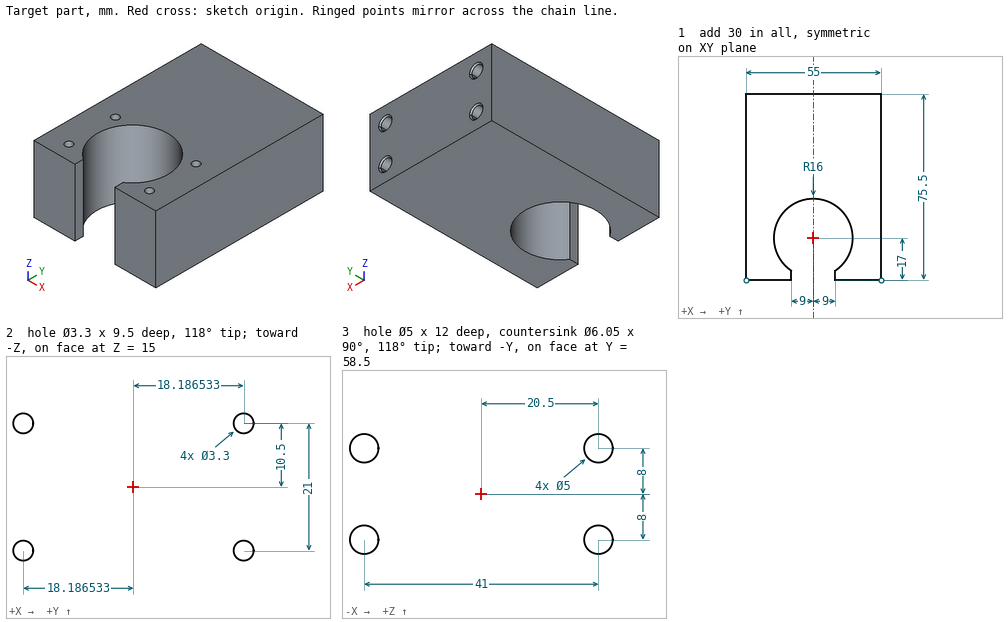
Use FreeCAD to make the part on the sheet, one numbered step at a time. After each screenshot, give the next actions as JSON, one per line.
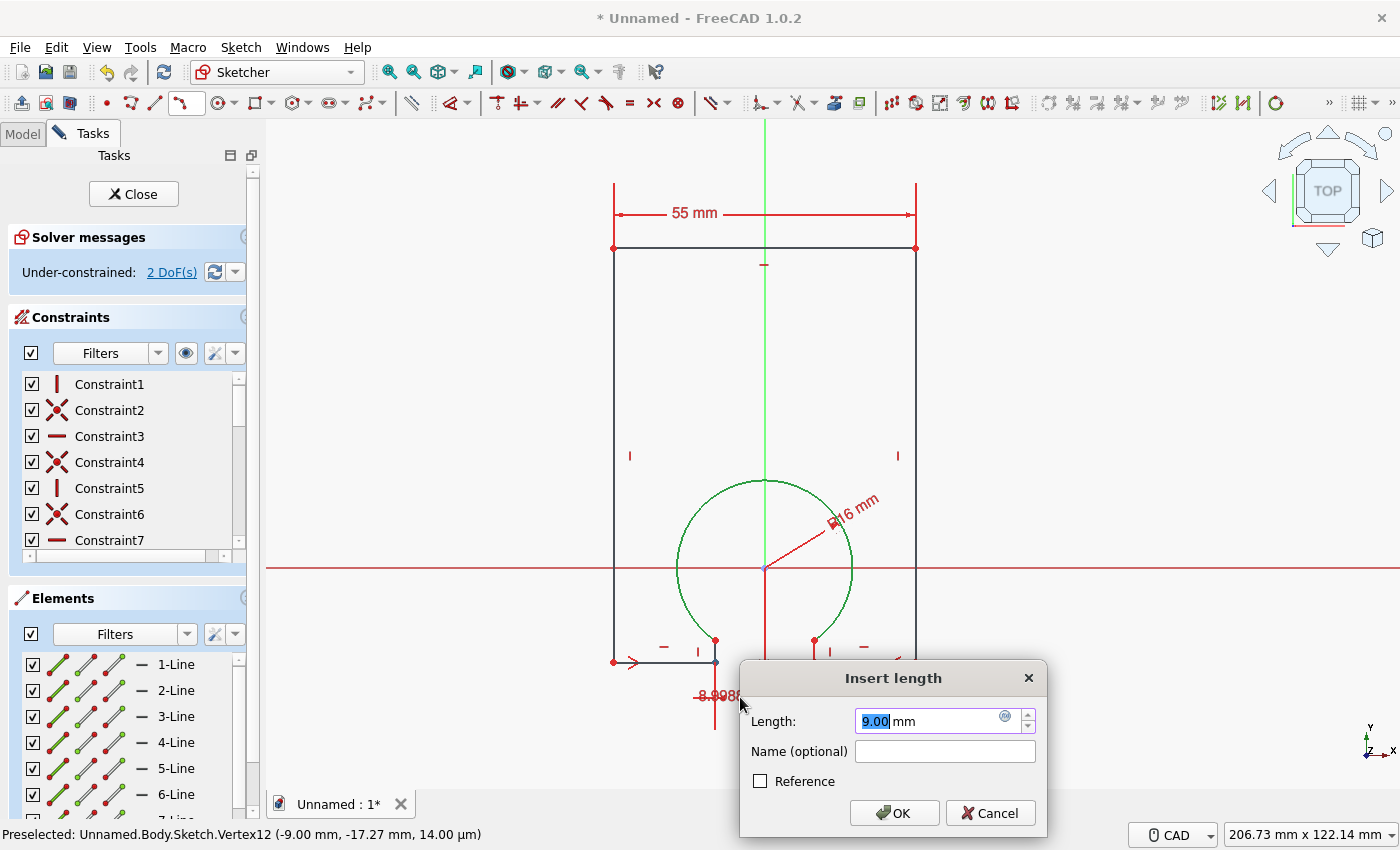
{"action": "type", "text": "9"}
{"action": "key", "text": "Return"}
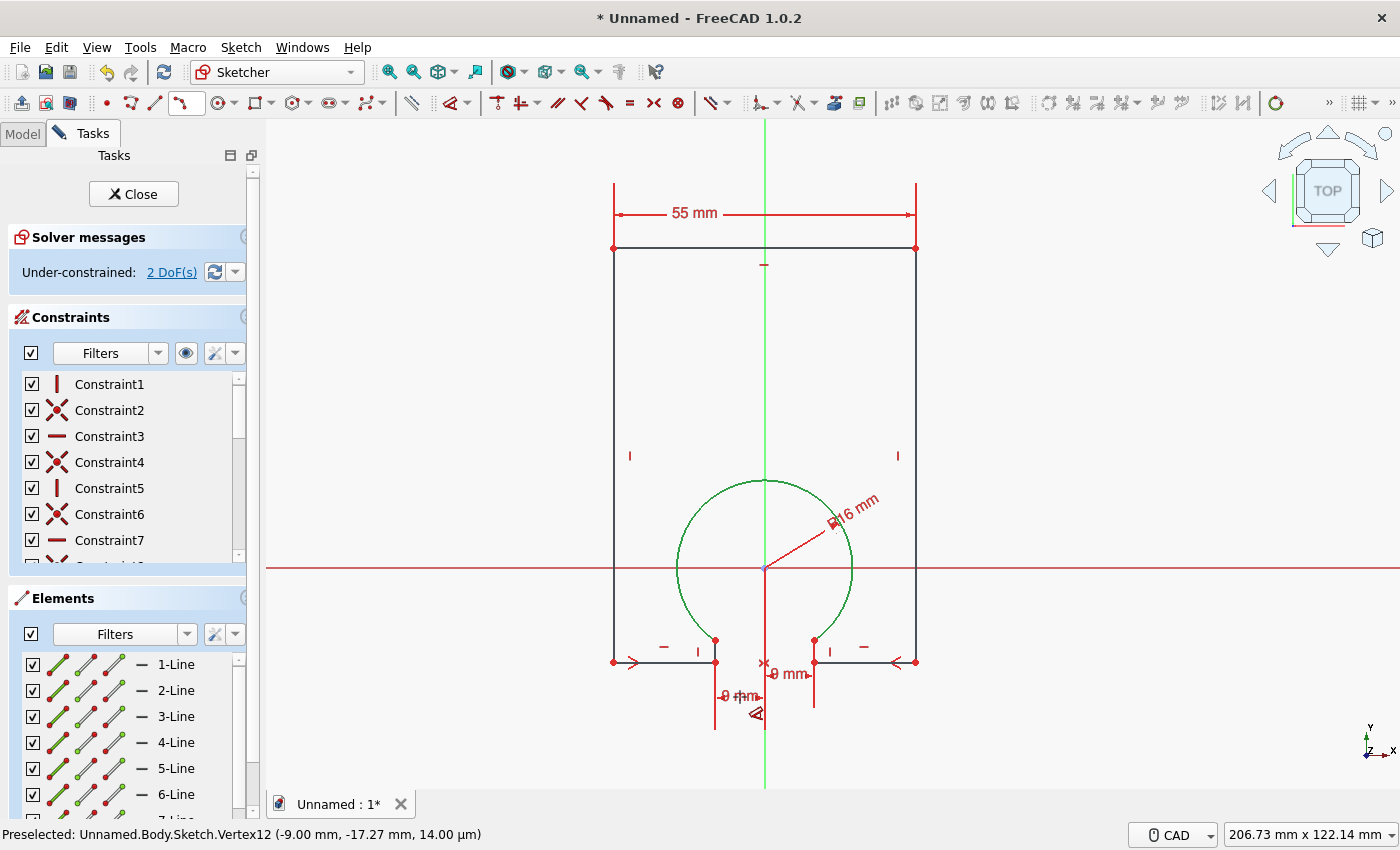
{"action": "left_click", "coordinate": [814, 663]}
{"action": "left_click", "coordinate": [848, 637]}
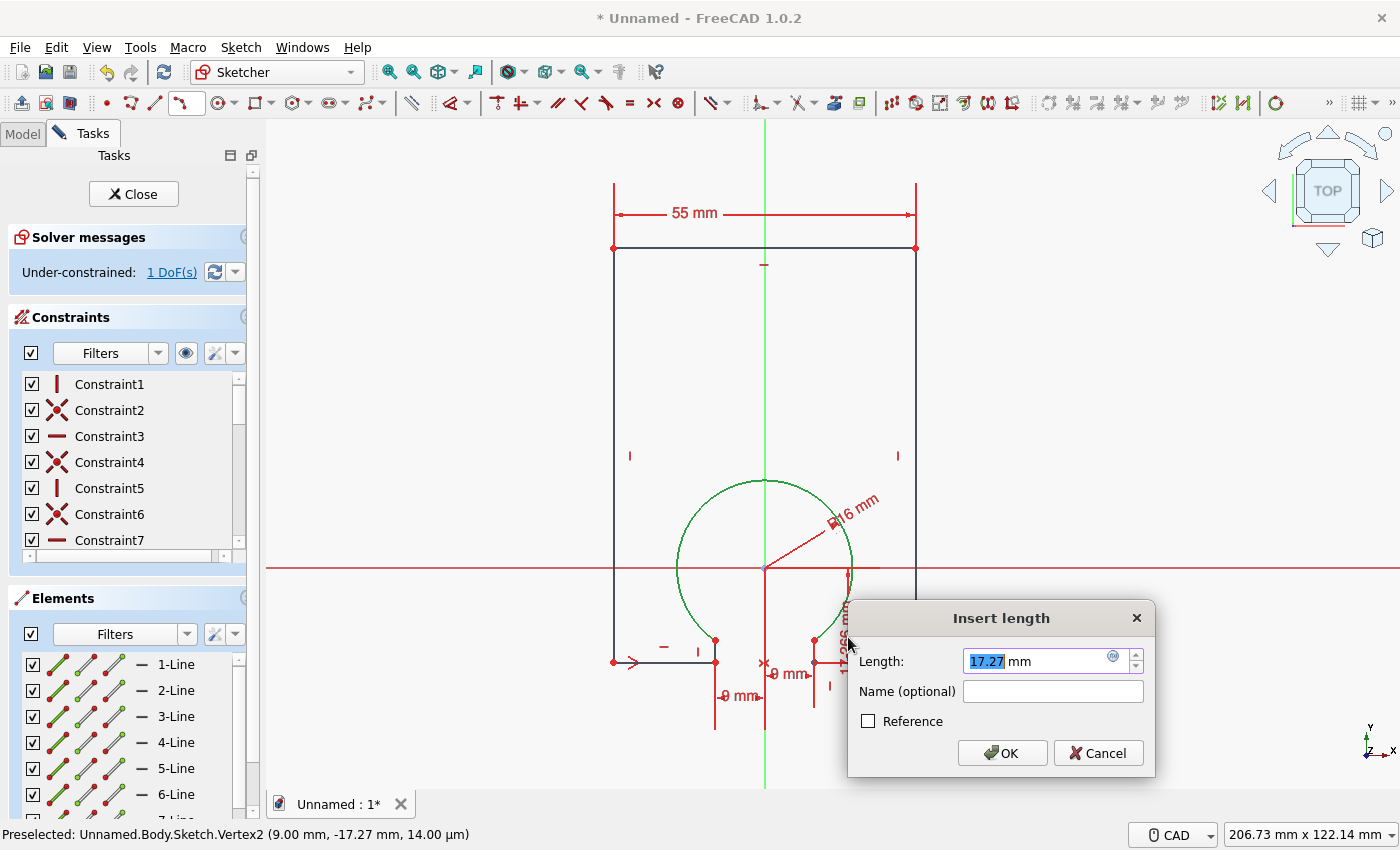
{"action": "type", "text": "17"}
{"action": "key", "text": "Return"}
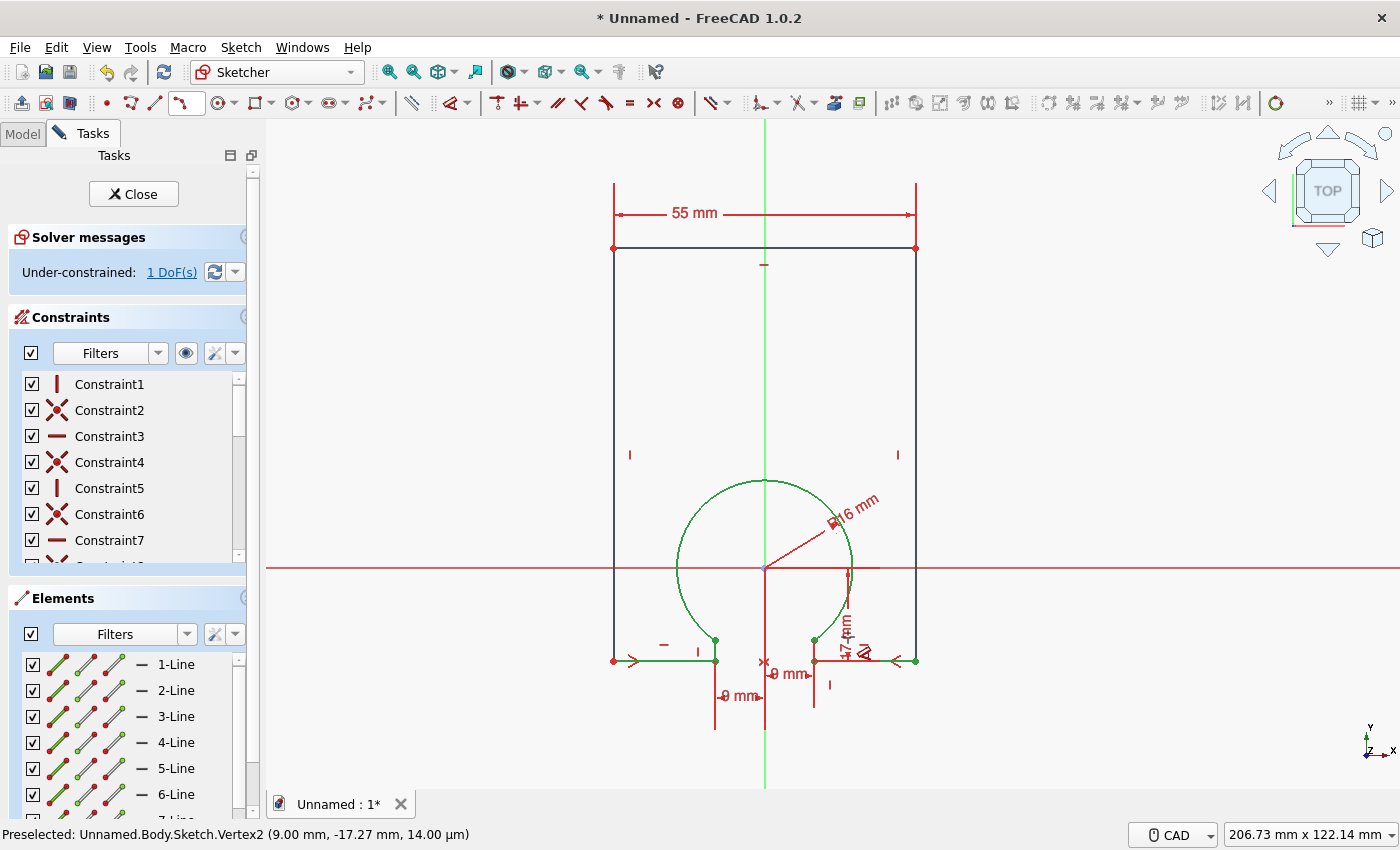
{"action": "left_click", "coordinate": [916, 537]}
{"action": "left_click", "coordinate": [950, 455]}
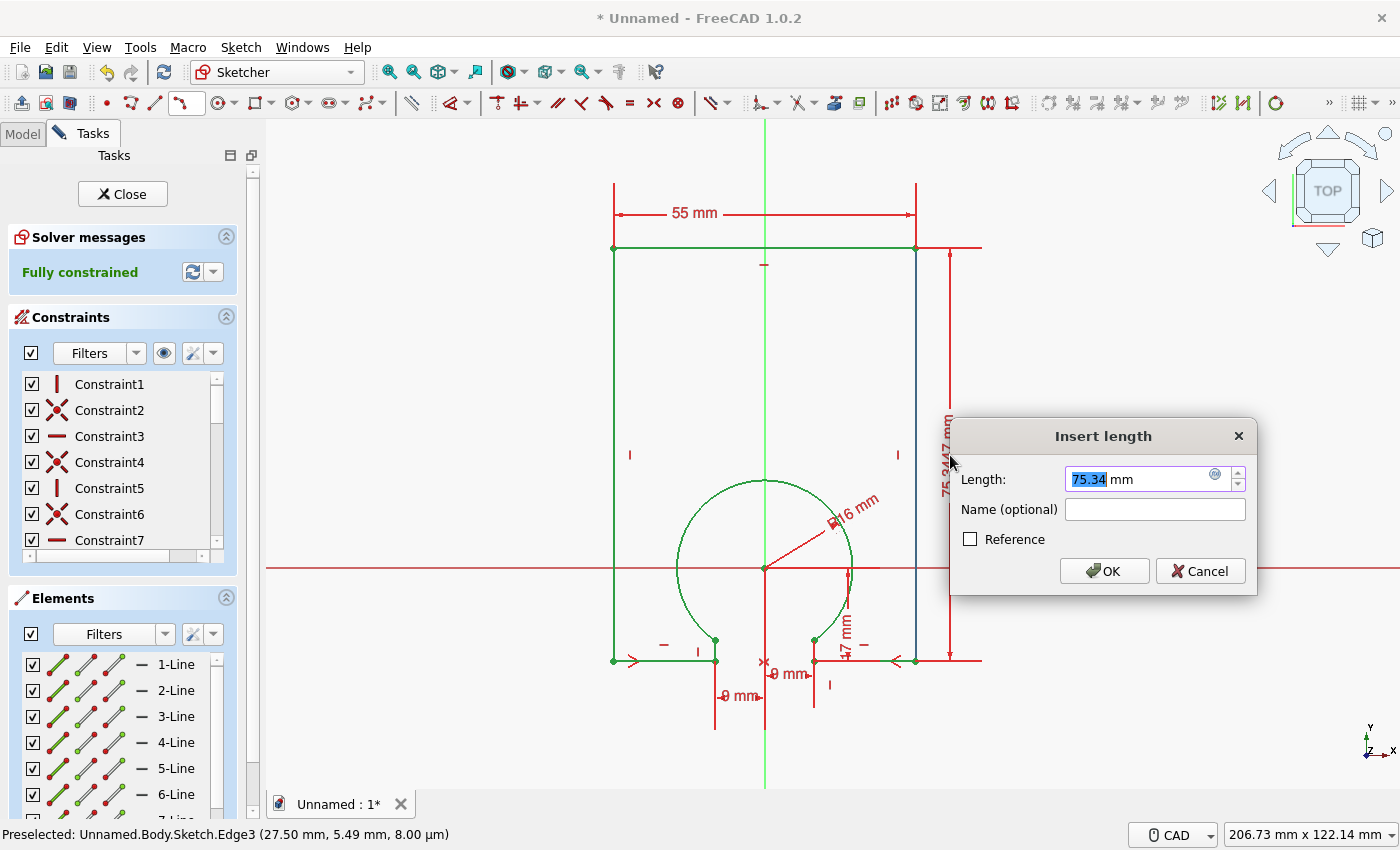
{"action": "type", "text": "75.5"}
{"action": "key", "text": "Return"}
{"action": "key", "text": "Escape"}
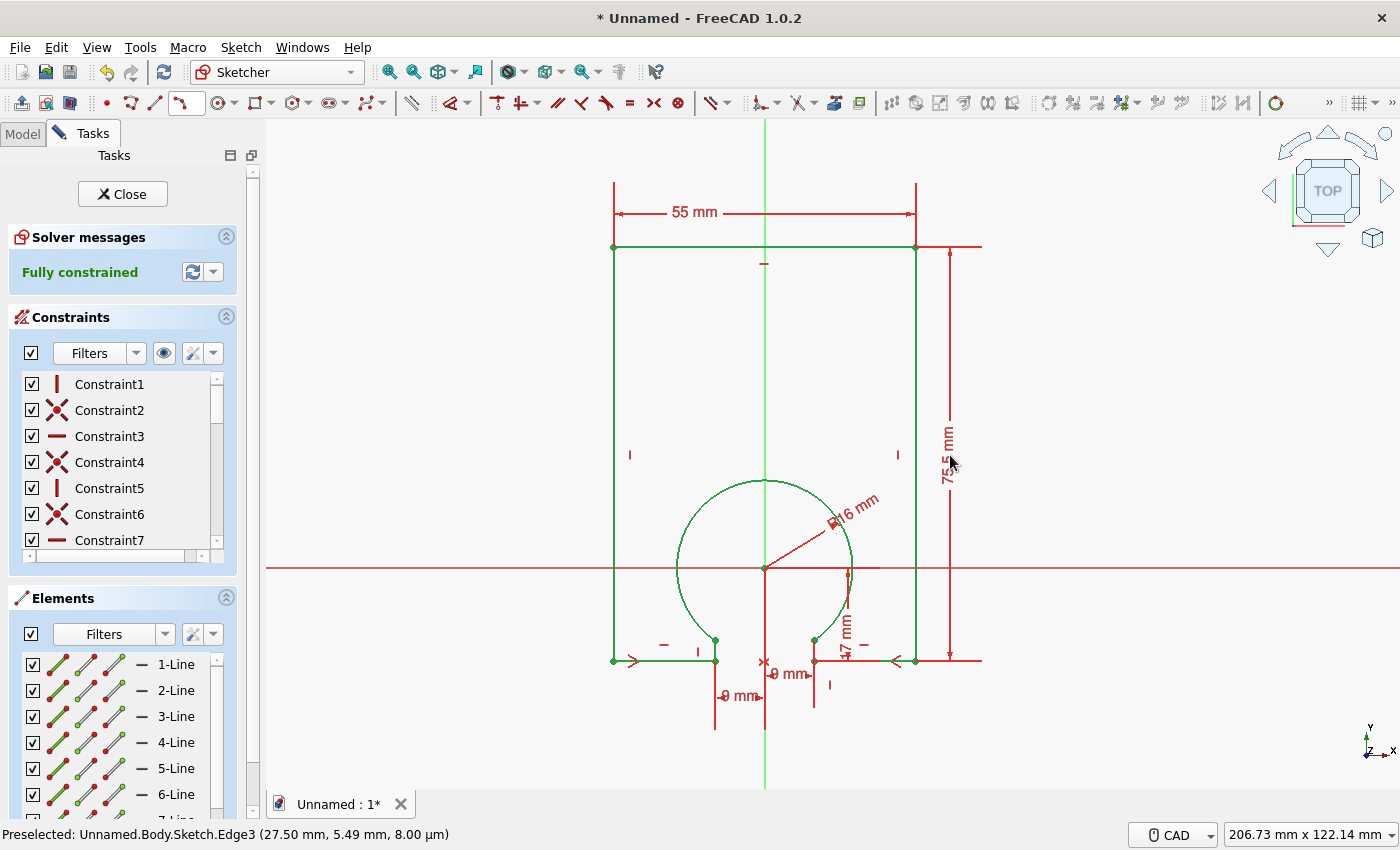
{"action": "left_click", "coordinate": [123, 194]}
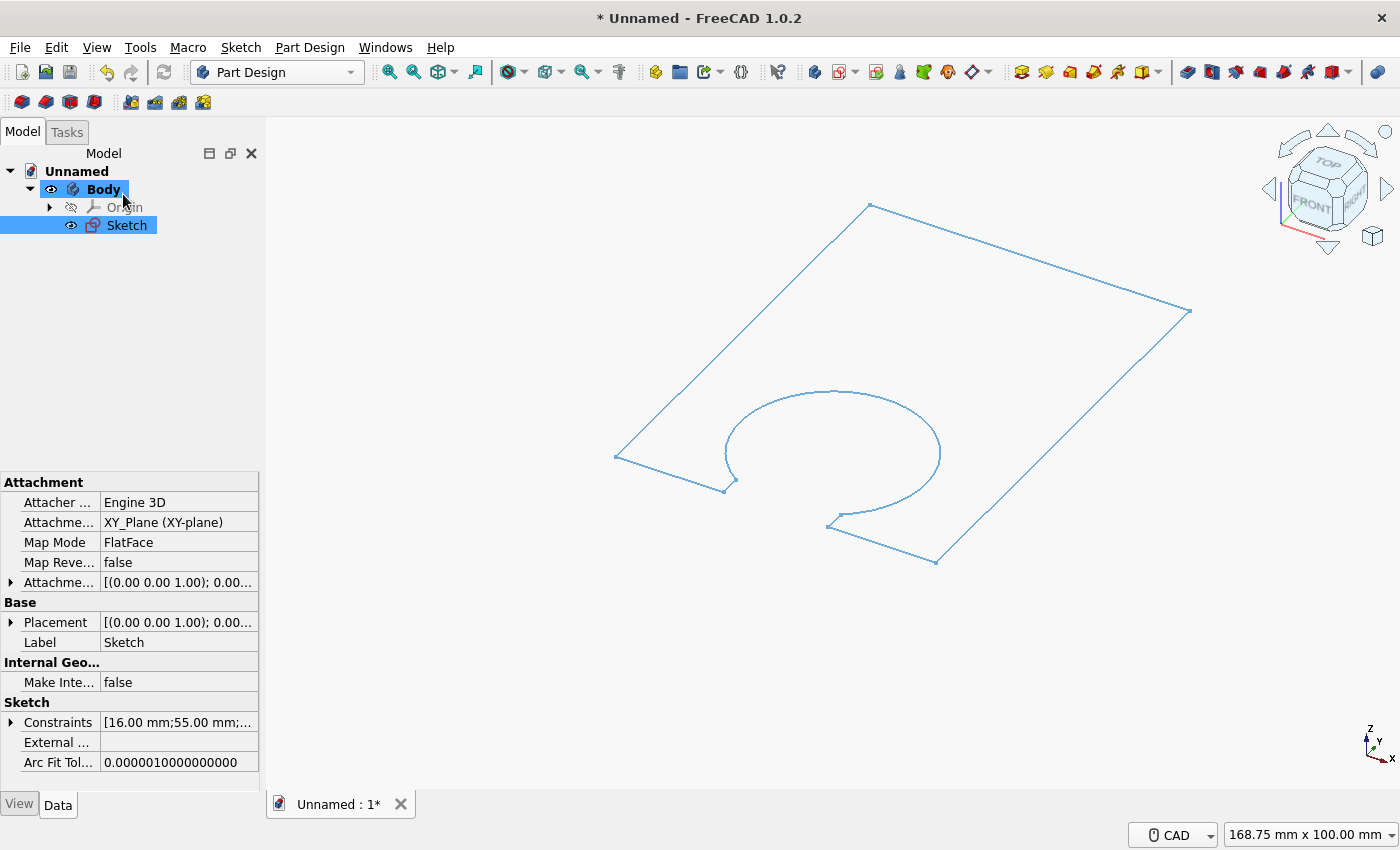
{"action": "left_click", "coordinate": [1022, 72]}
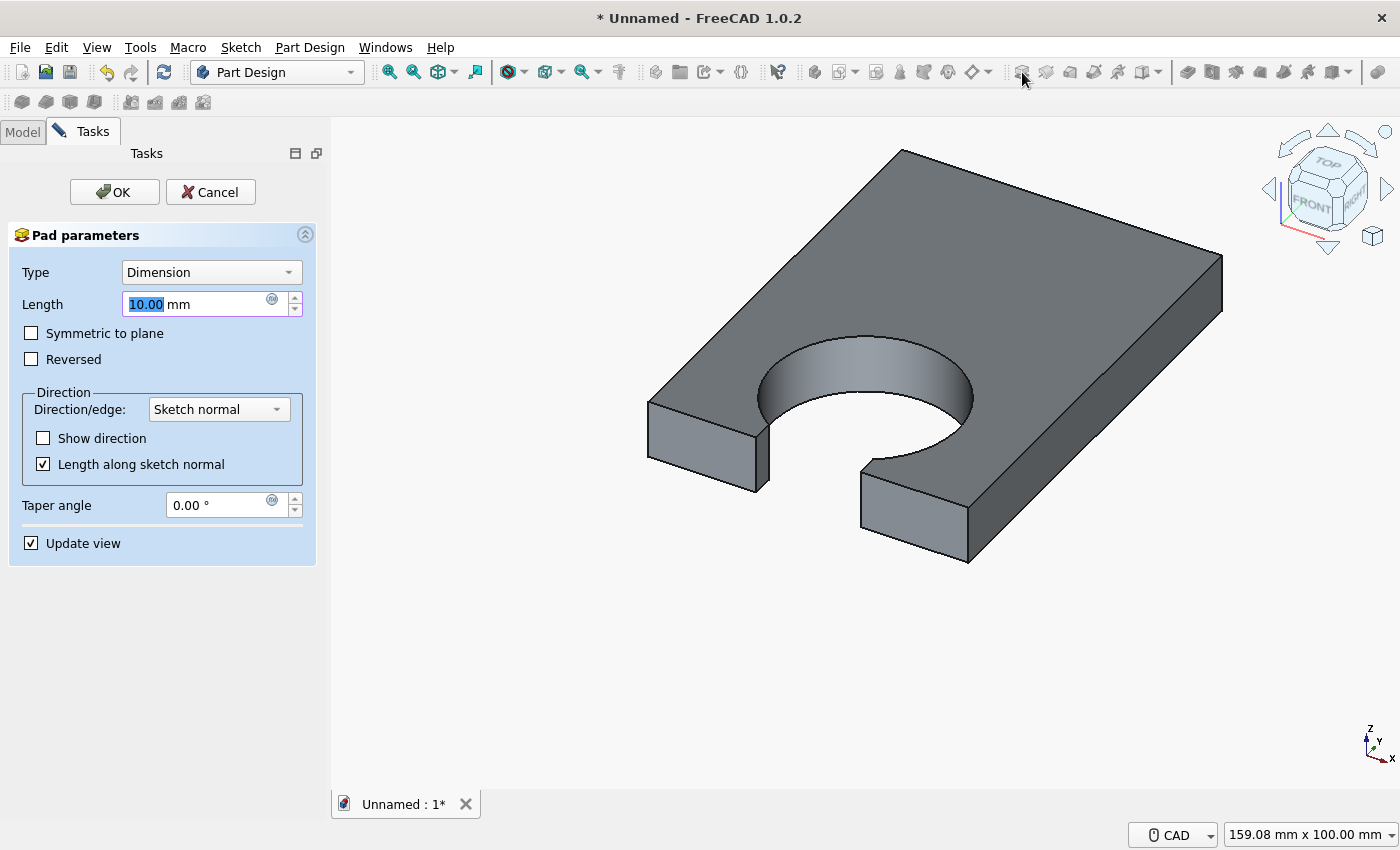
{"action": "type", "text": "30"}
{"action": "key", "text": "Tab"}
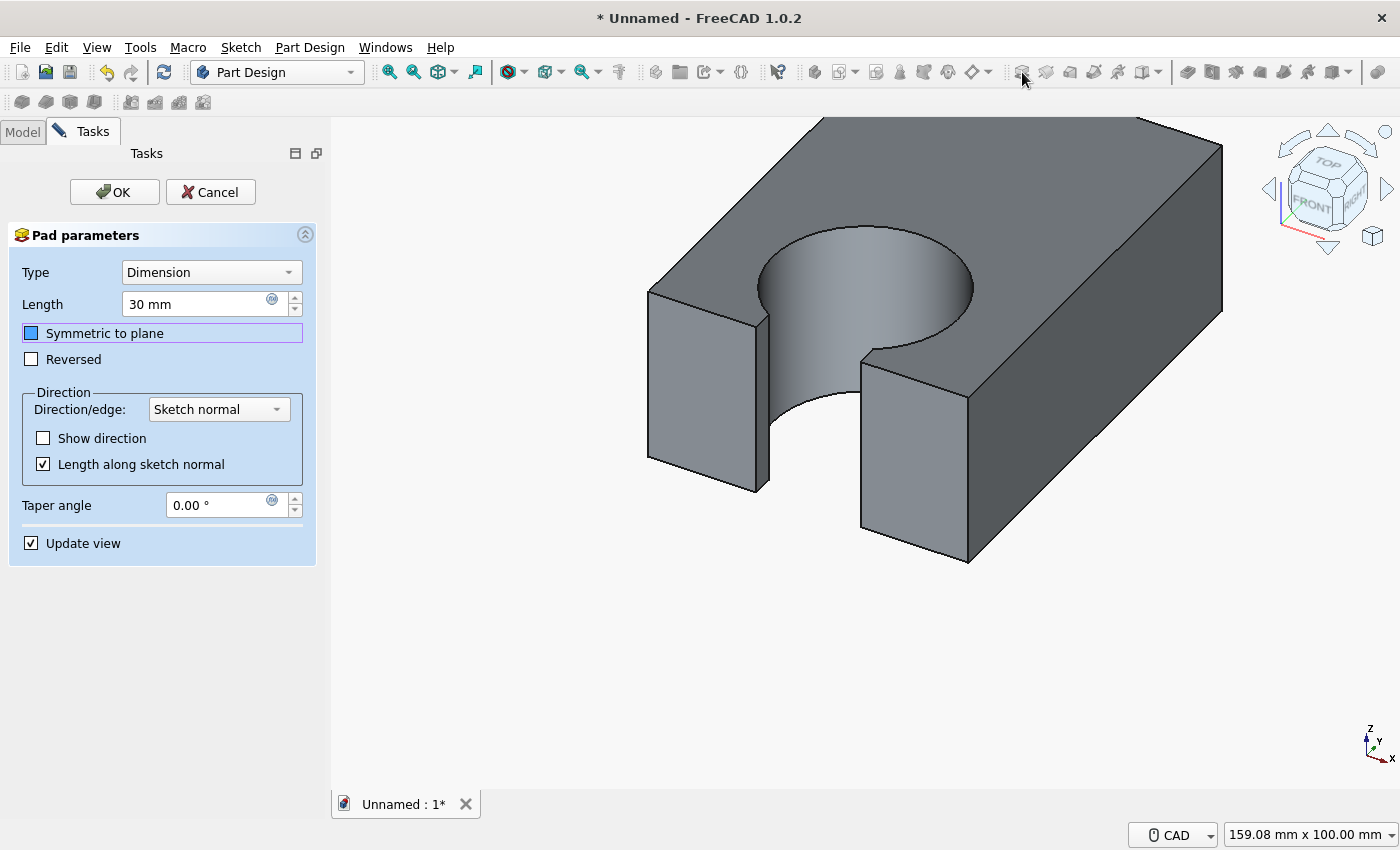
{"action": "left_click", "coordinate": [30, 333]}